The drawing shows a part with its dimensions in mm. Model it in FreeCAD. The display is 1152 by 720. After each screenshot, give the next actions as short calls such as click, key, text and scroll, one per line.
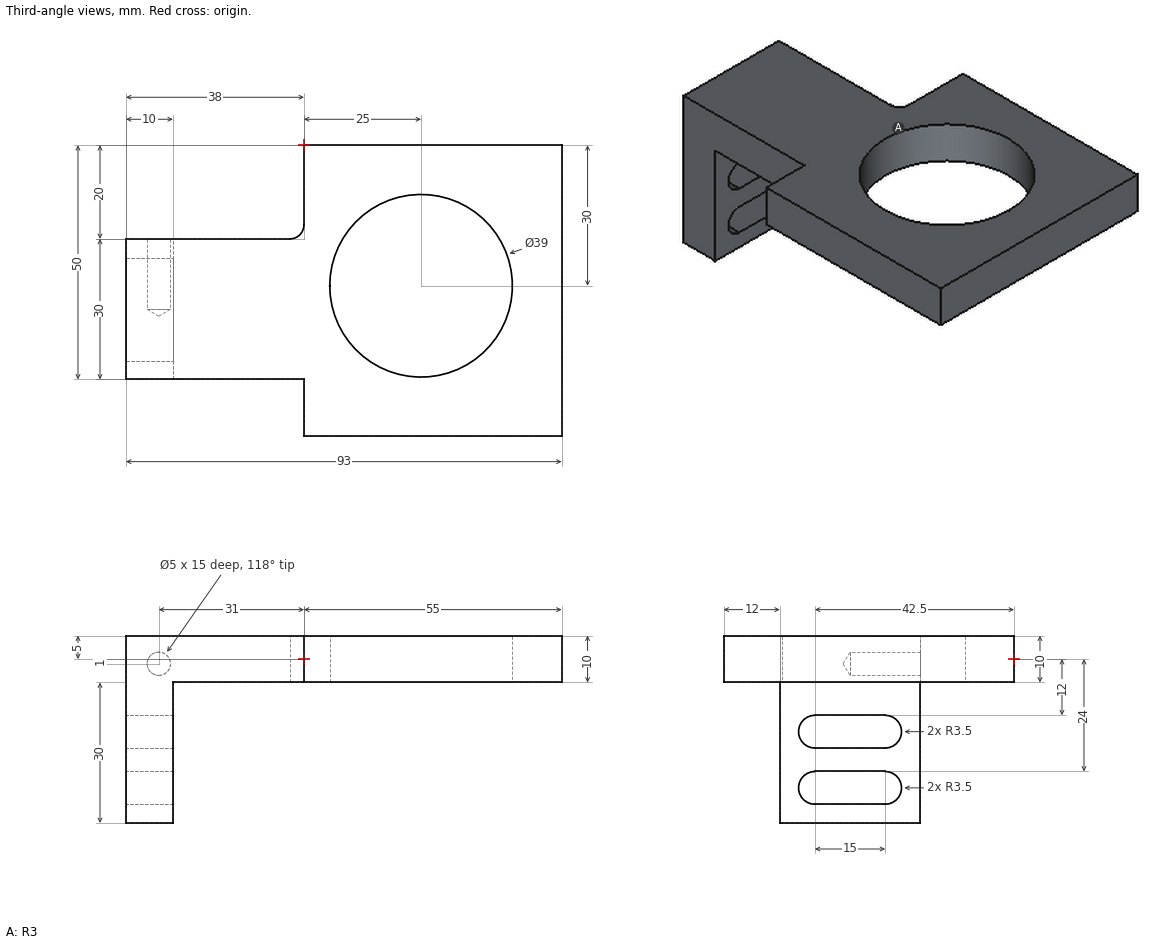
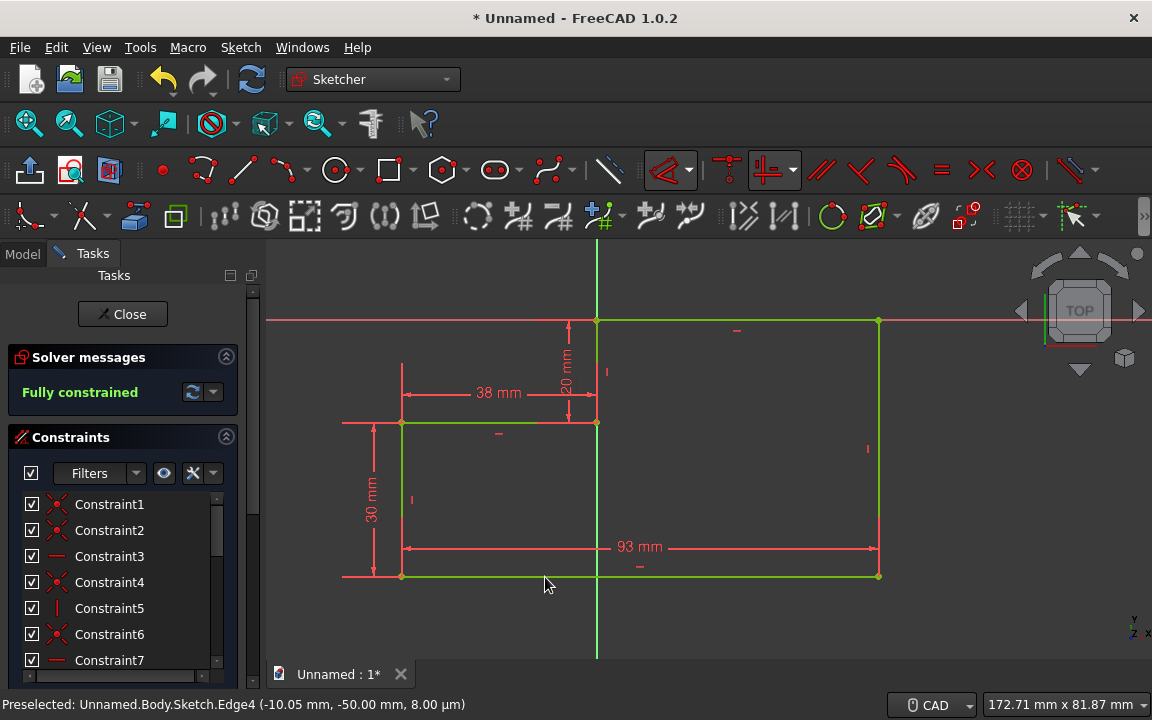
click(123, 314)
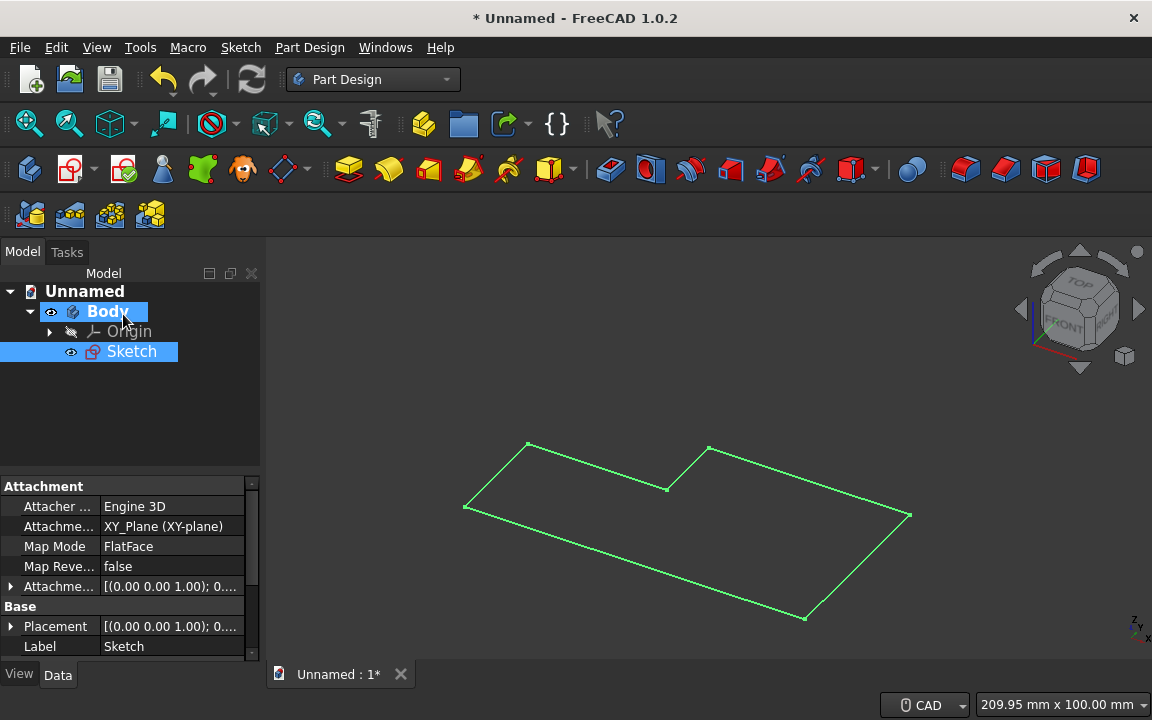
click(350, 170)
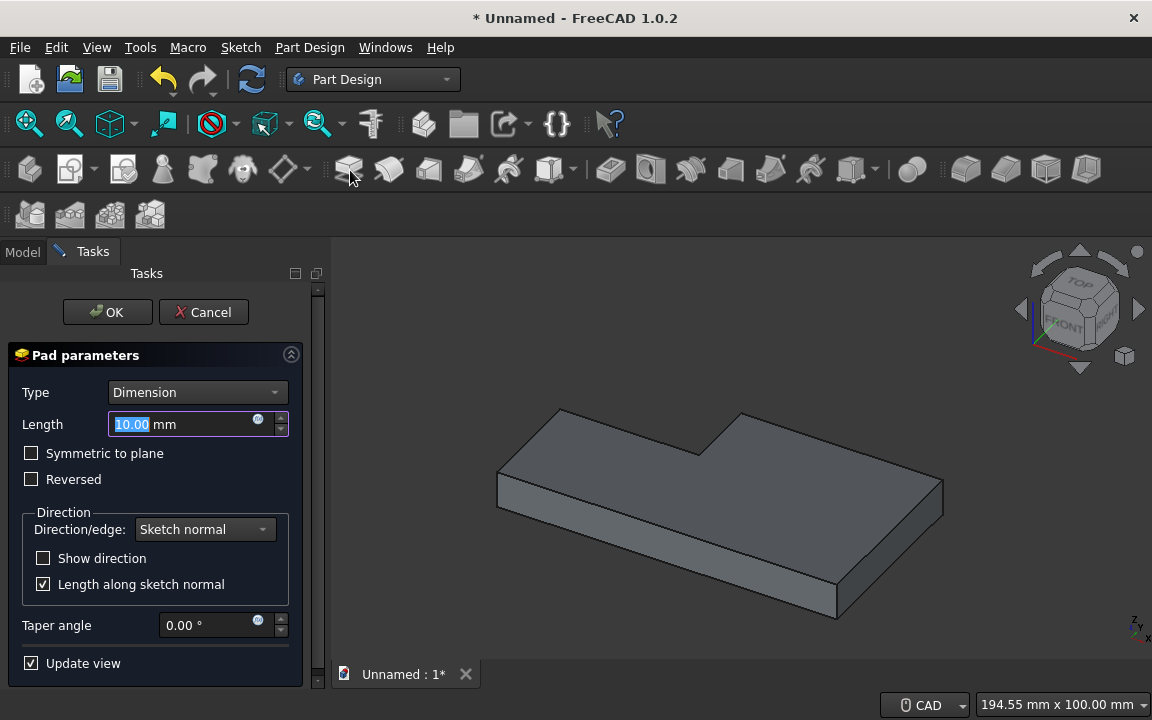
text(10)
key(Tab)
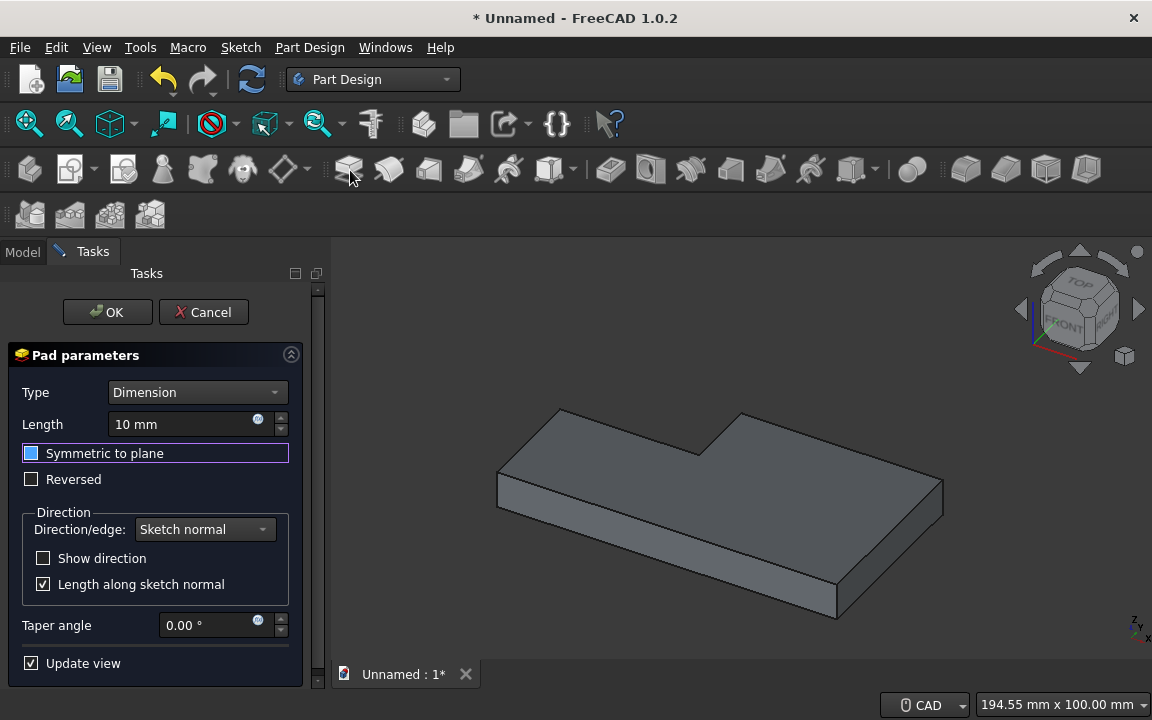
click(30, 453)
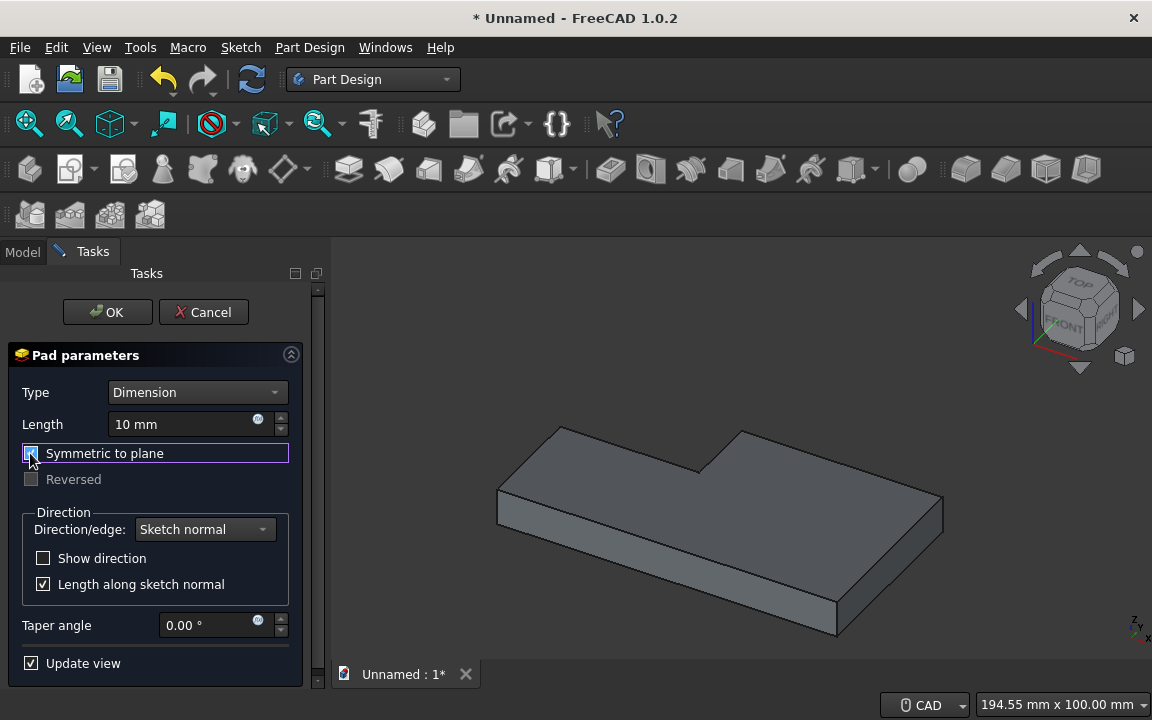
click(108, 312)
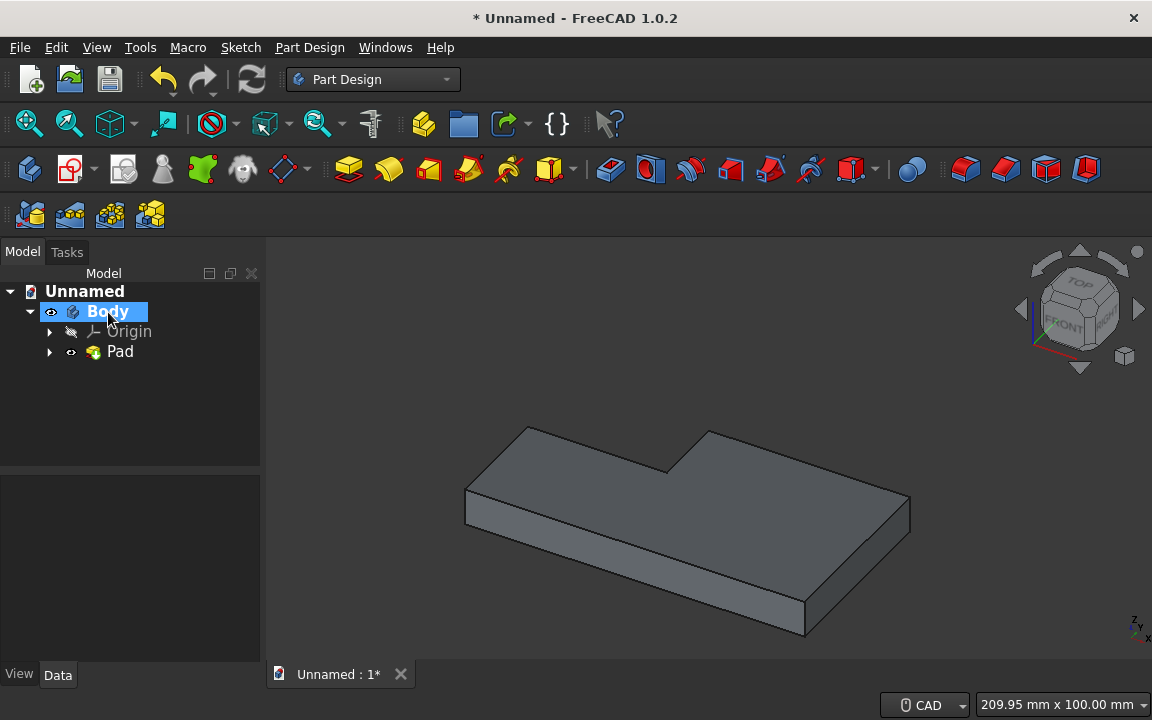
key(0)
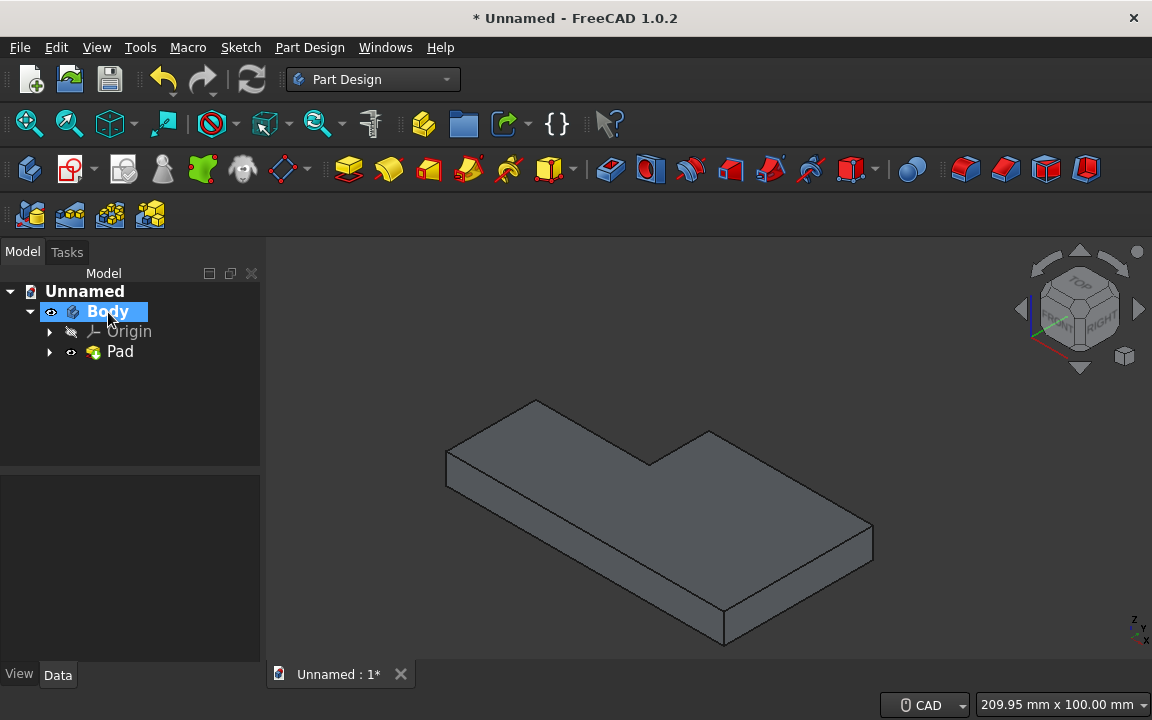
key(2)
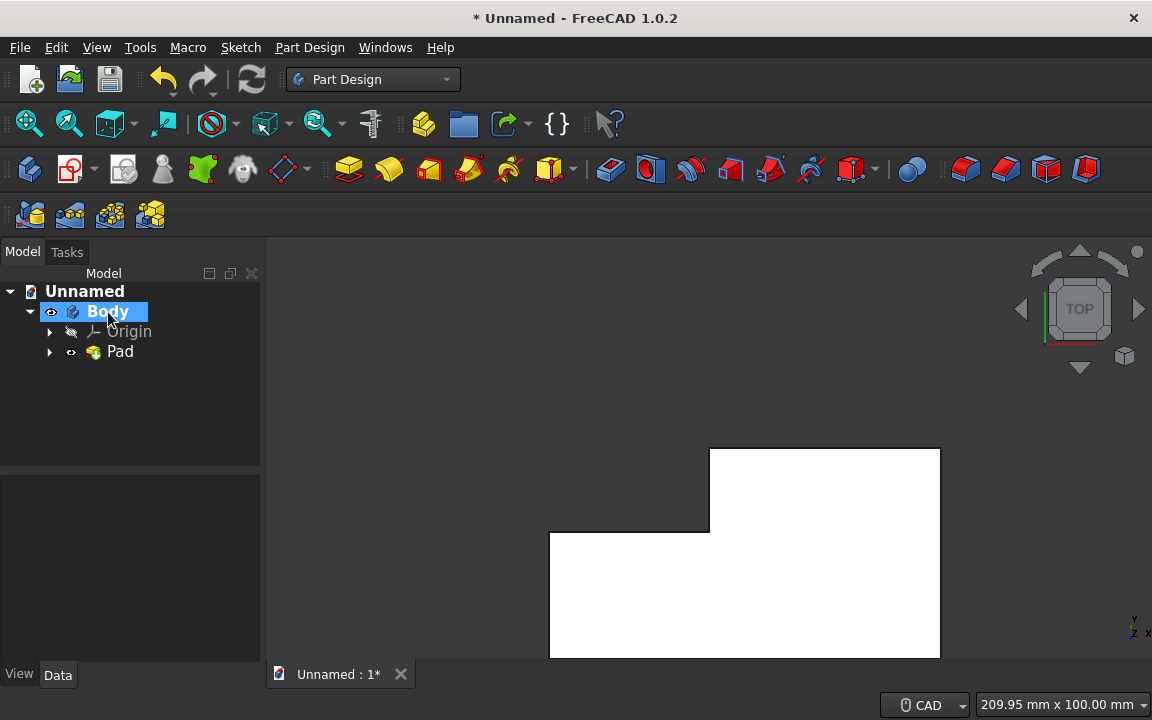
key(1)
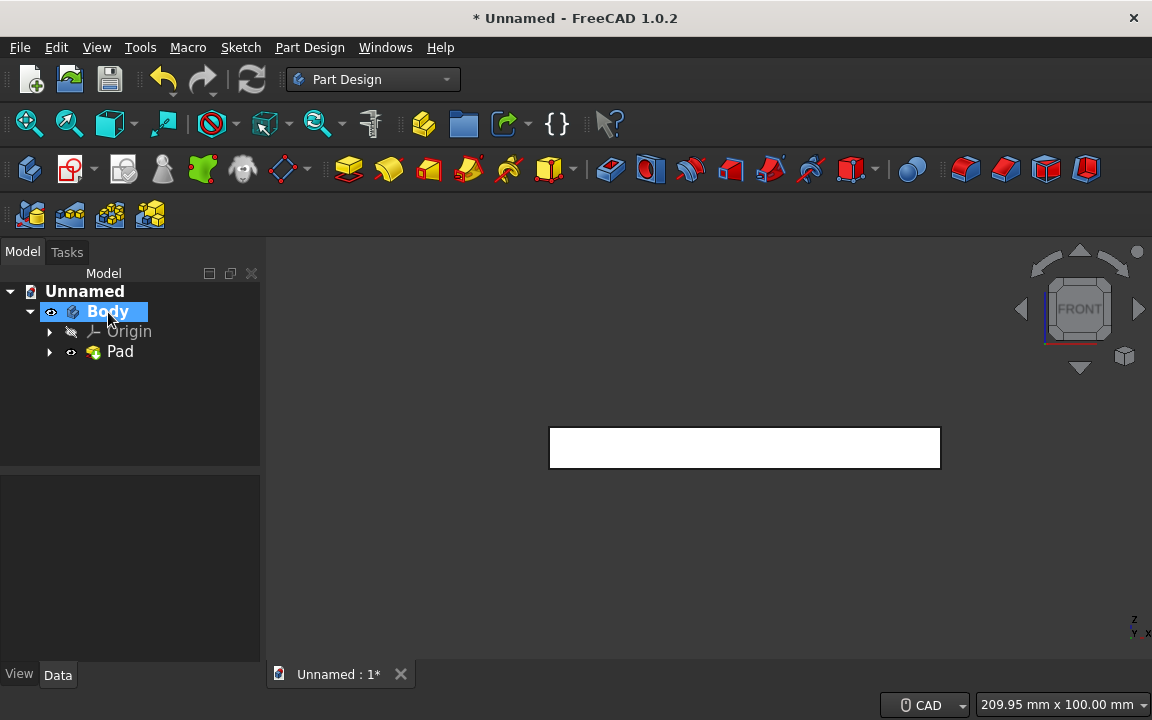
click(30, 124)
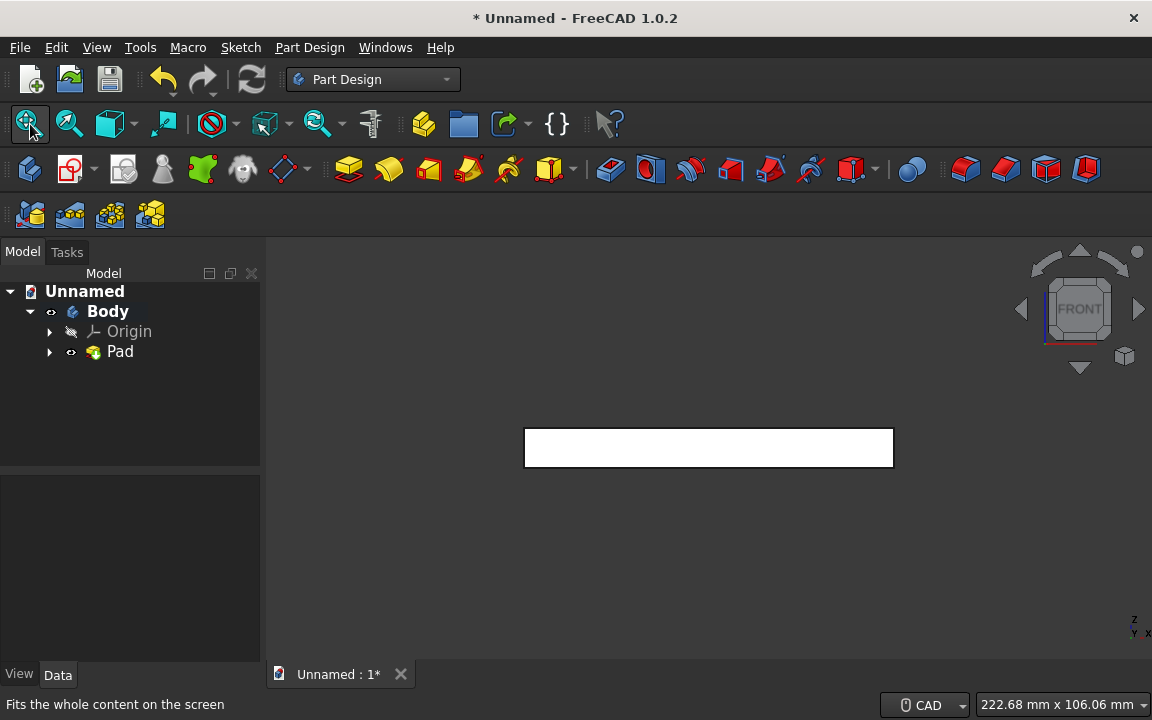
key(3)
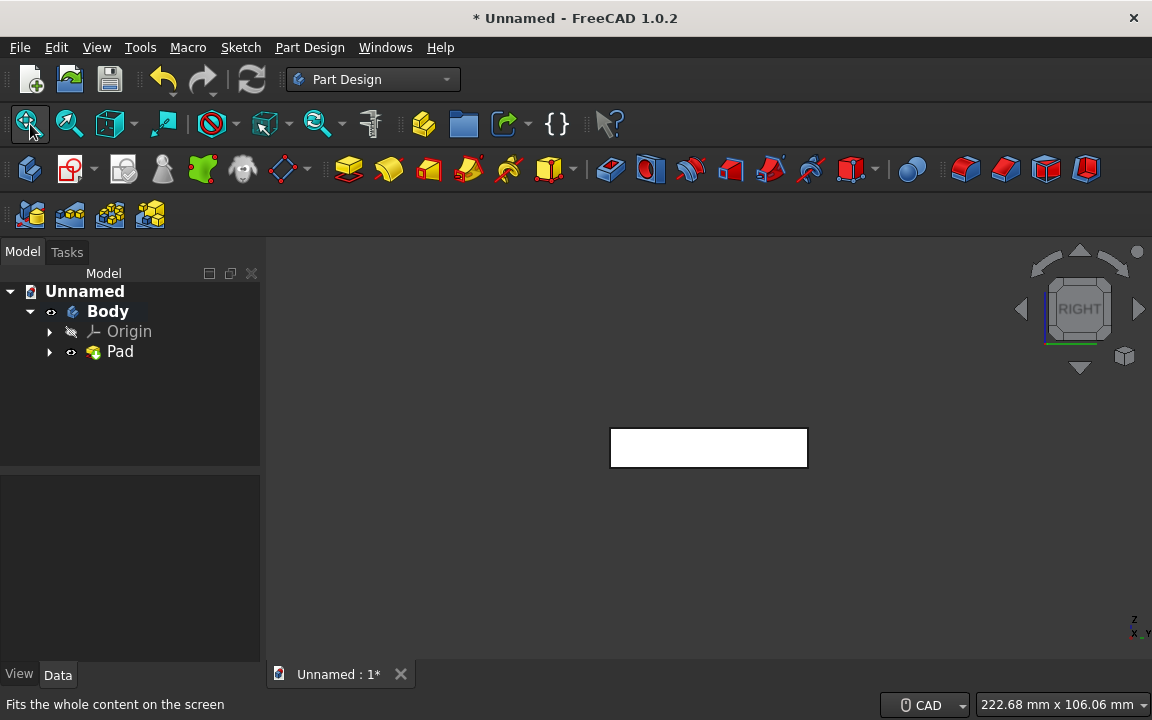
click(30, 124)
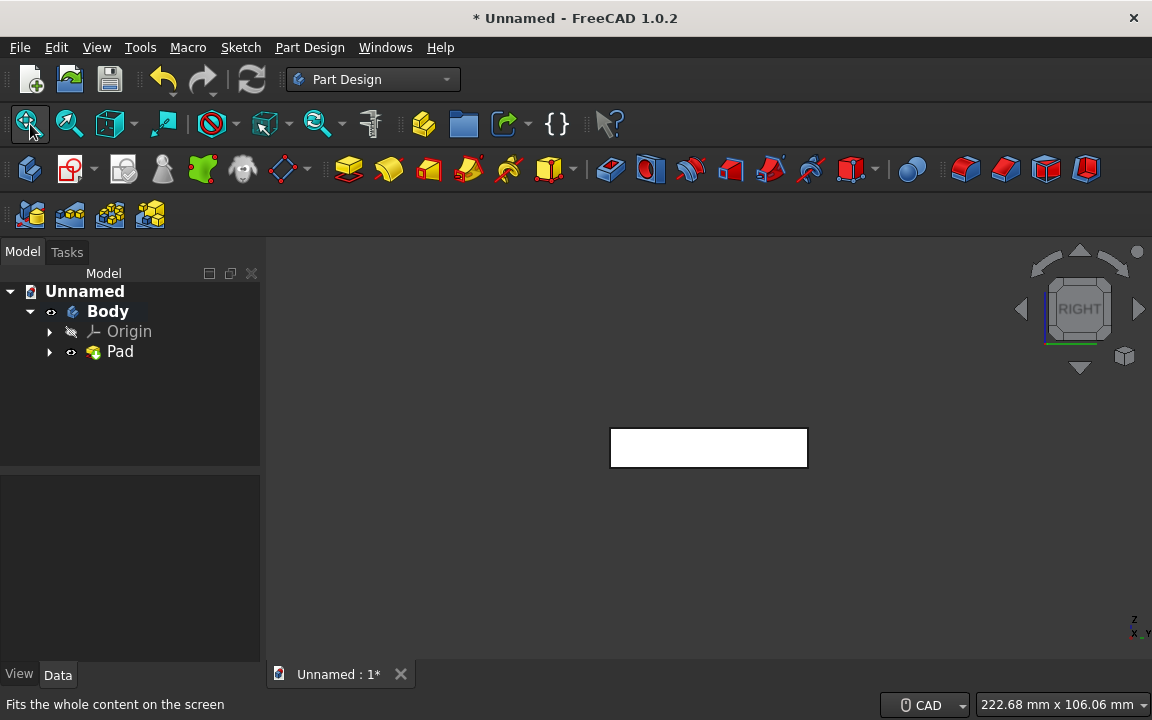
key(5)